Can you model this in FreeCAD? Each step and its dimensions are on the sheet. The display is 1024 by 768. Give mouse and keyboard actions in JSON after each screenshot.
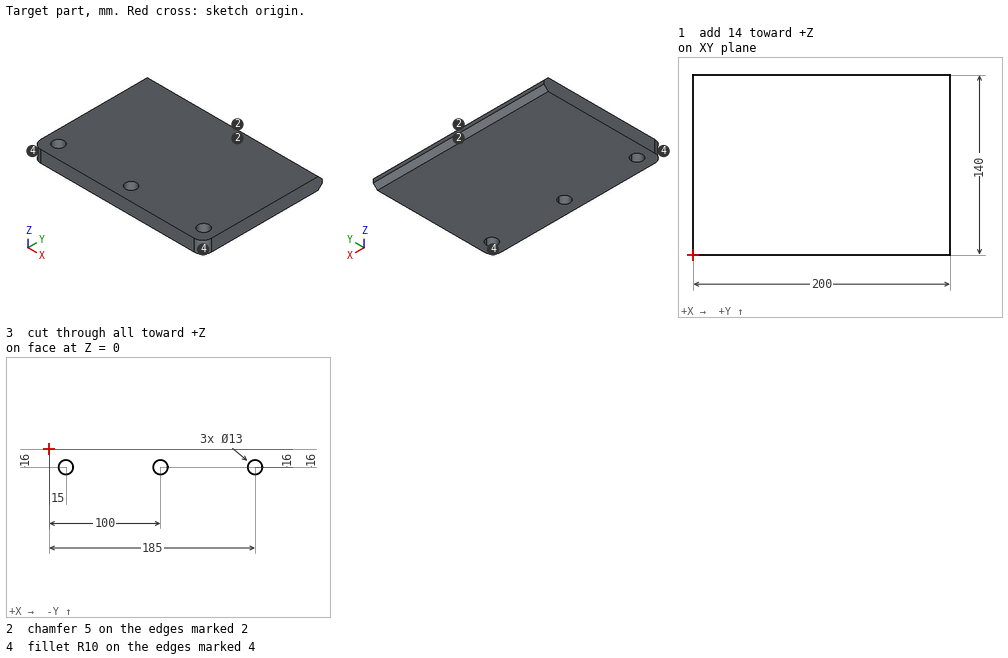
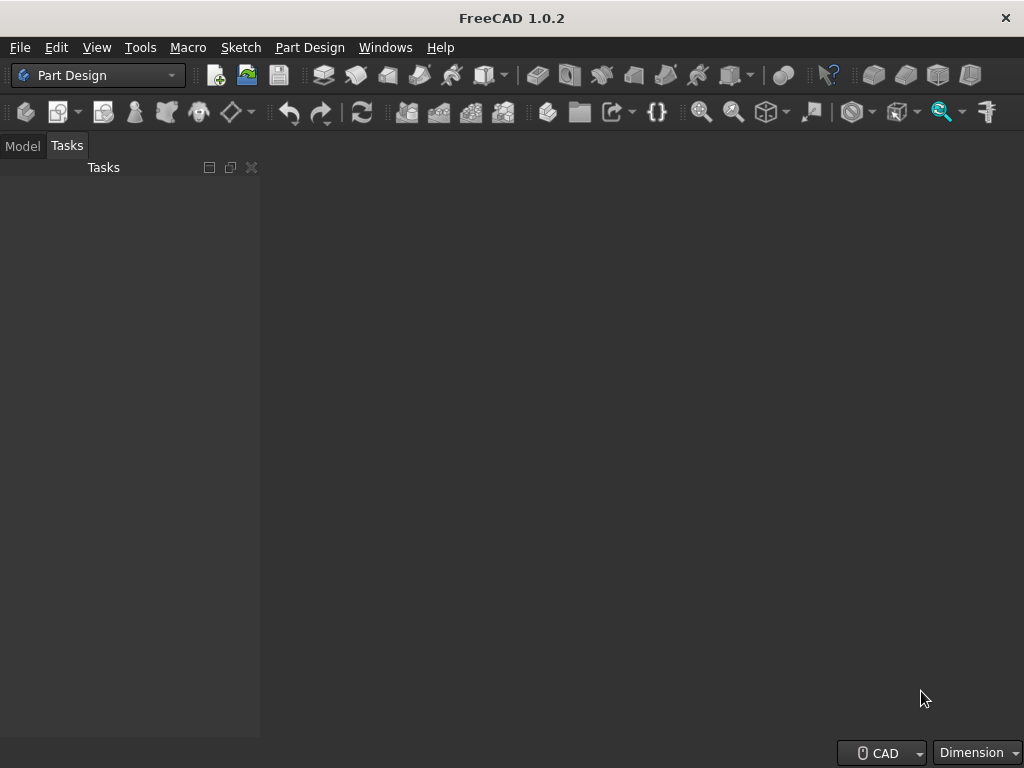
{"action": "left_click", "coordinate": [216, 76]}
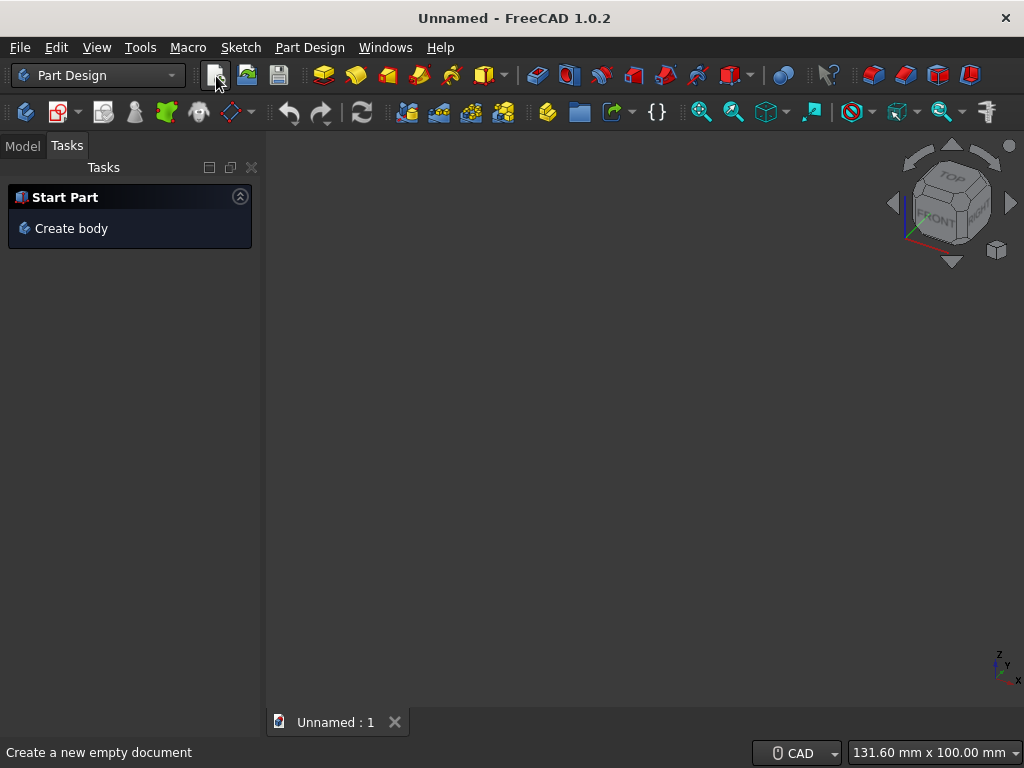
{"action": "left_click", "coordinate": [58, 112]}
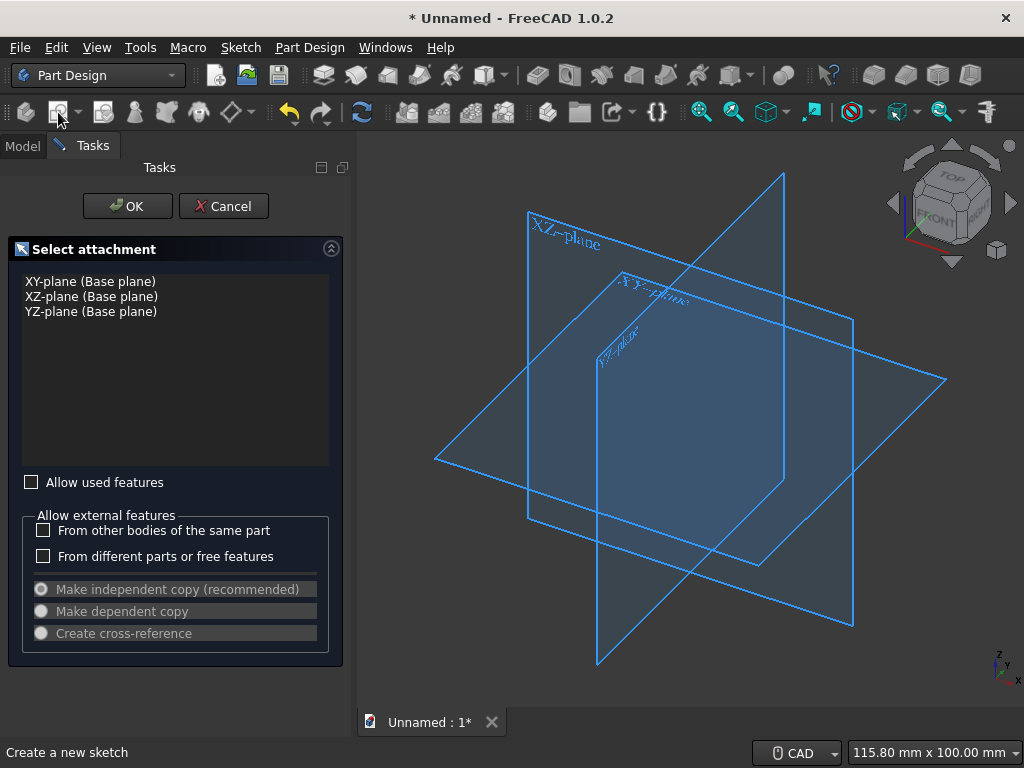
{"action": "left_click", "coordinate": [82, 282]}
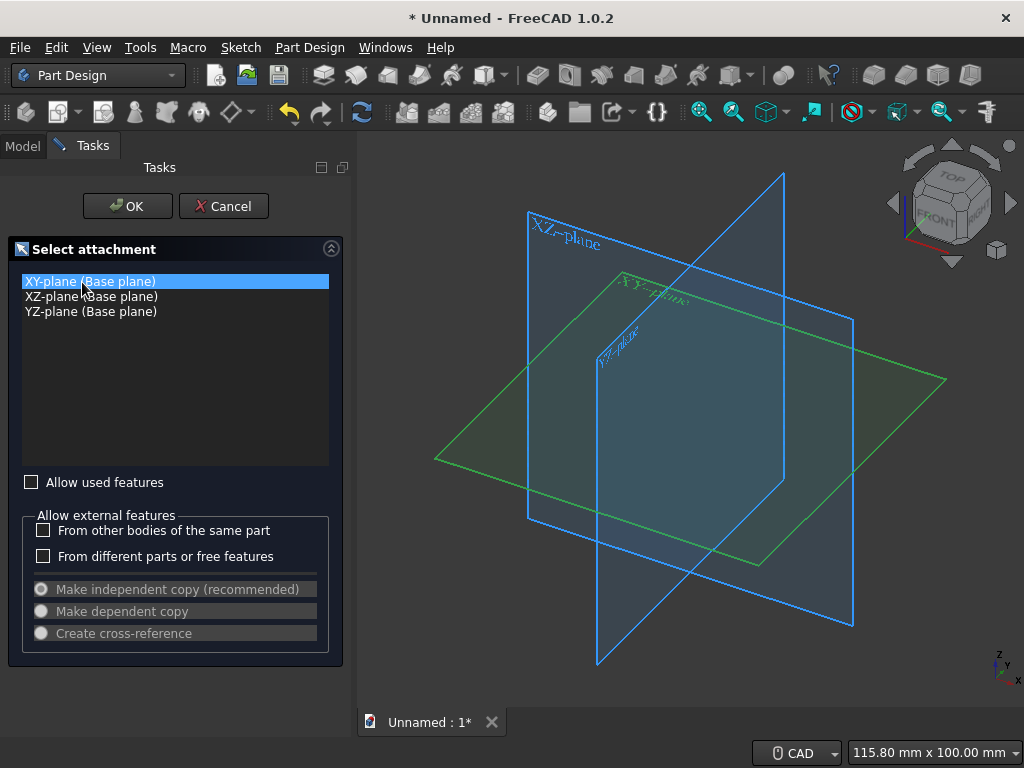
{"action": "left_click", "coordinate": [128, 206]}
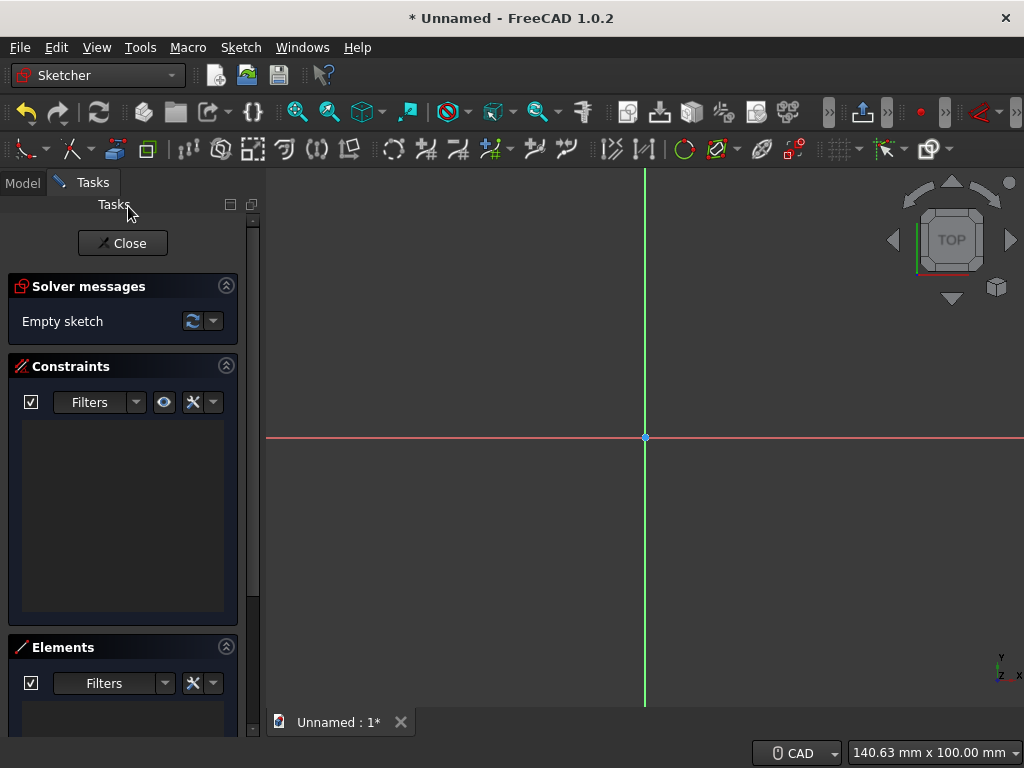
{"action": "scroll", "coordinate": [294, 657], "scroll_direction": "down", "scroll_amount": 5}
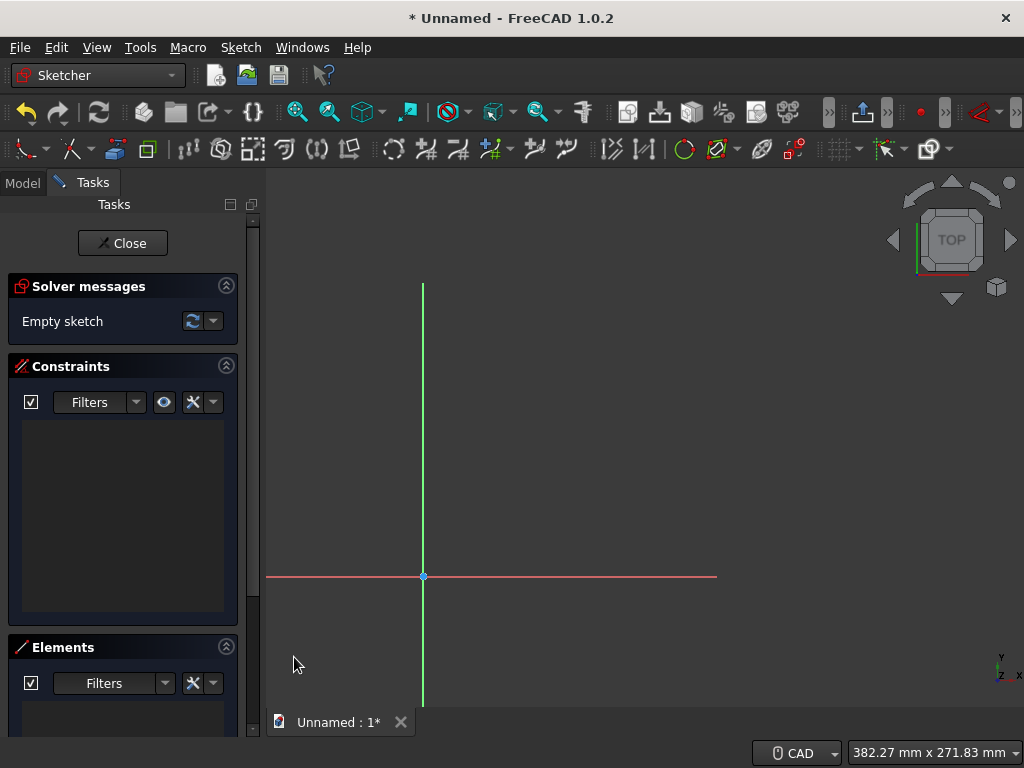
{"action": "key", "text": "g r"}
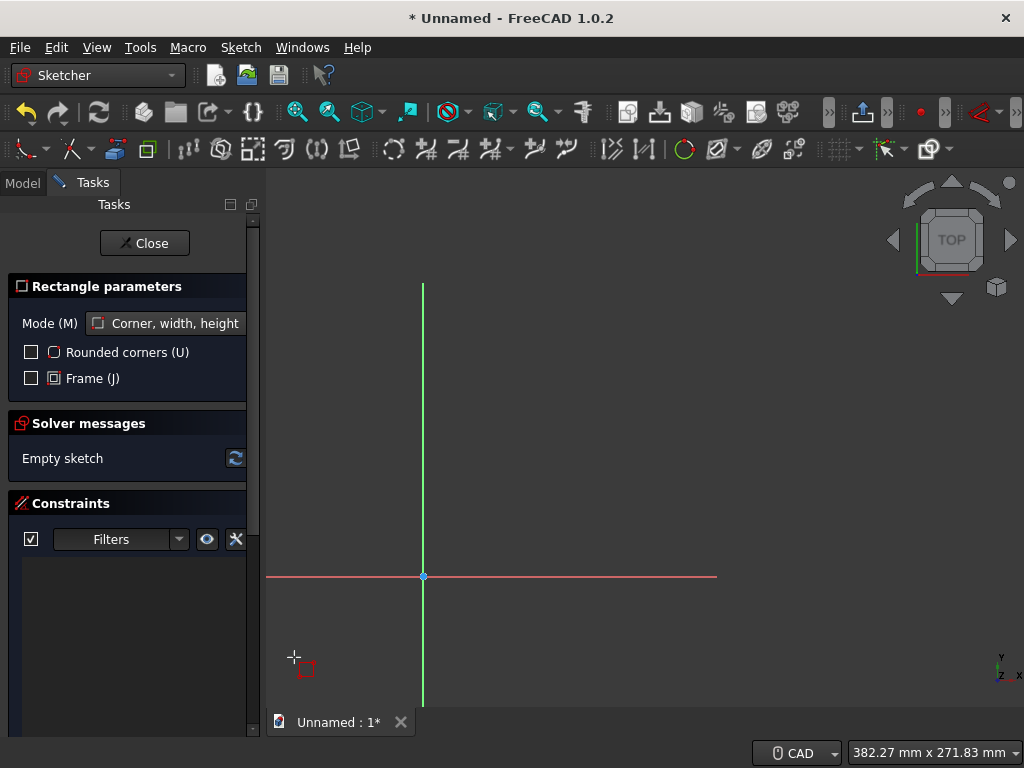
{"action": "left_click", "coordinate": [423, 577]}
{"action": "left_click", "coordinate": [820, 299]}
{"action": "key", "text": "Escape"}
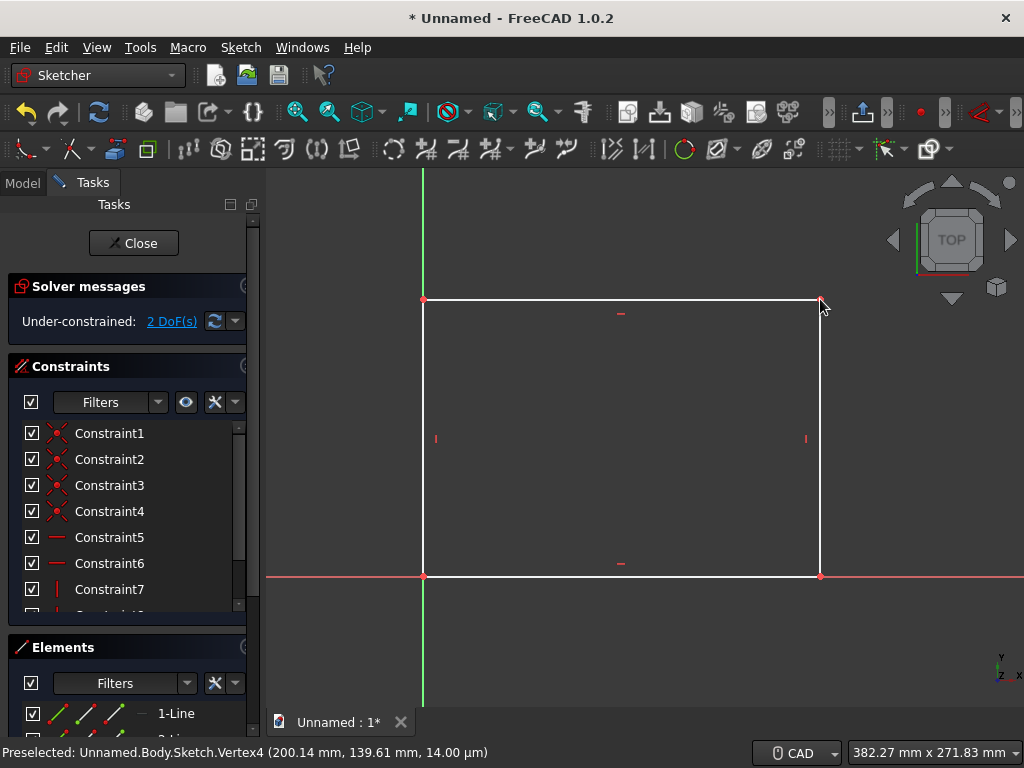
{"action": "left_click", "coordinate": [980, 112]}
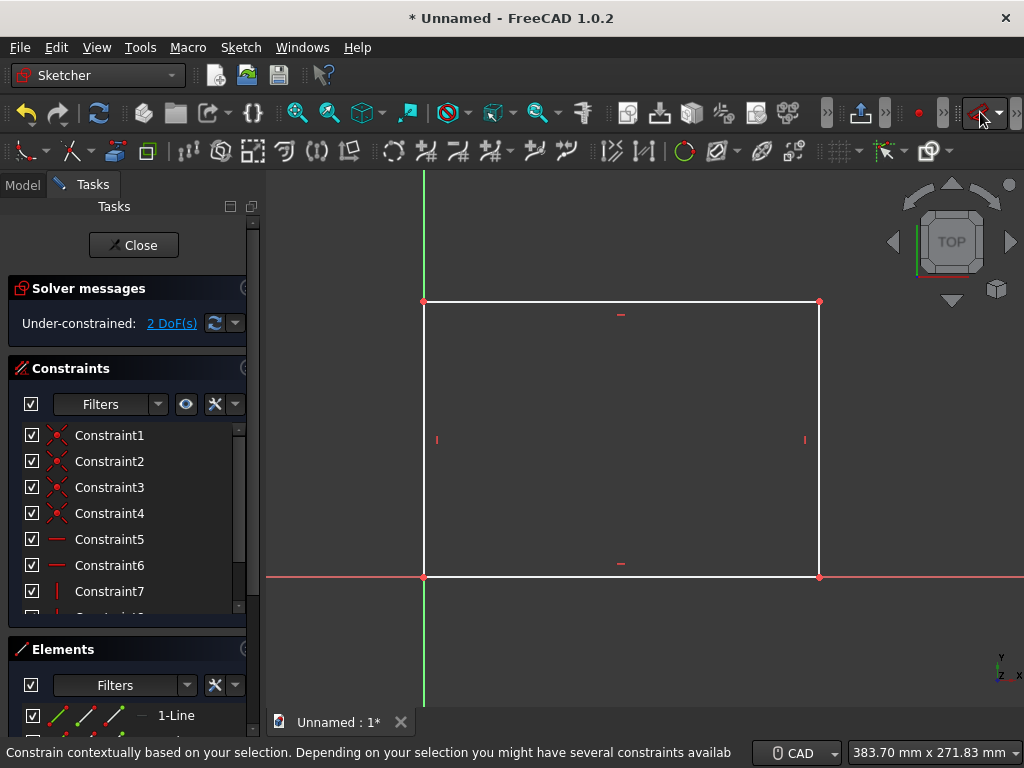
{"action": "left_click", "coordinate": [543, 577]}
{"action": "left_click", "coordinate": [622, 611]}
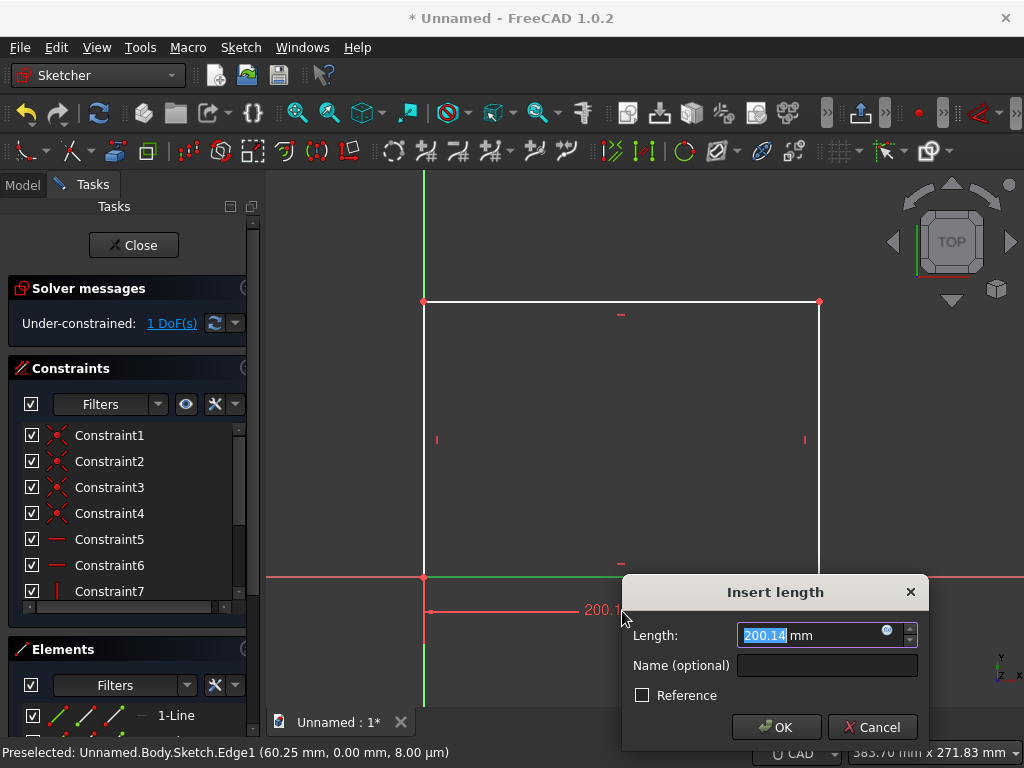
{"action": "type", "text": "200"}
{"action": "key", "text": "Return"}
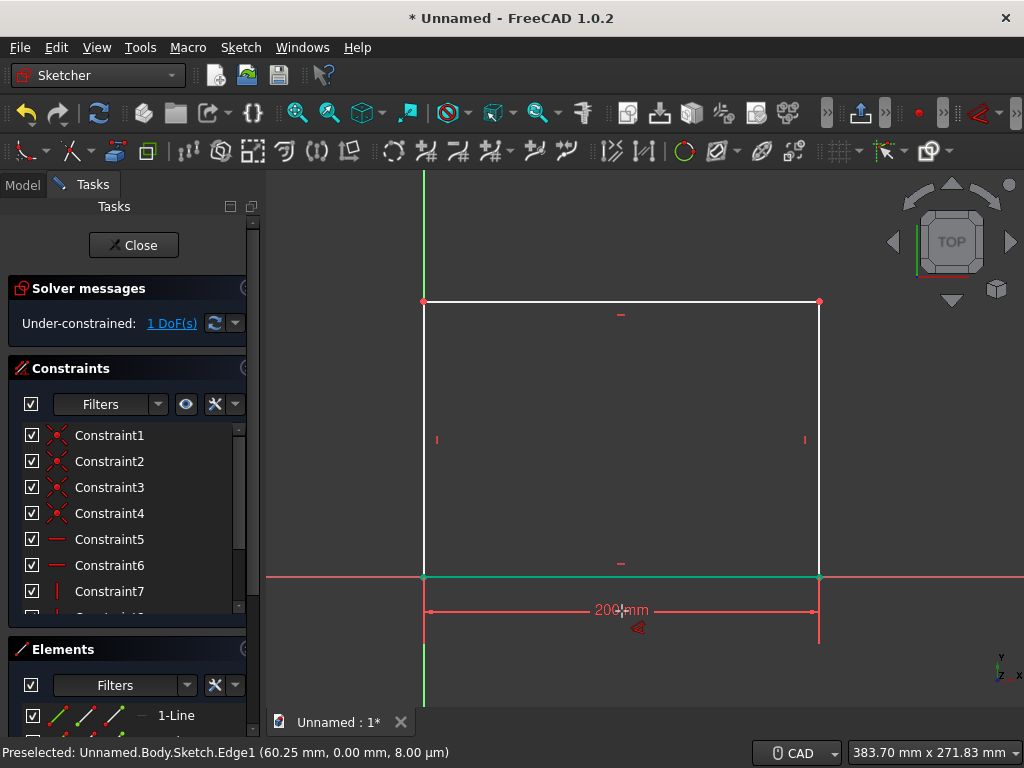
{"action": "left_click", "coordinate": [819, 495]}
{"action": "left_click", "coordinate": [853, 439]}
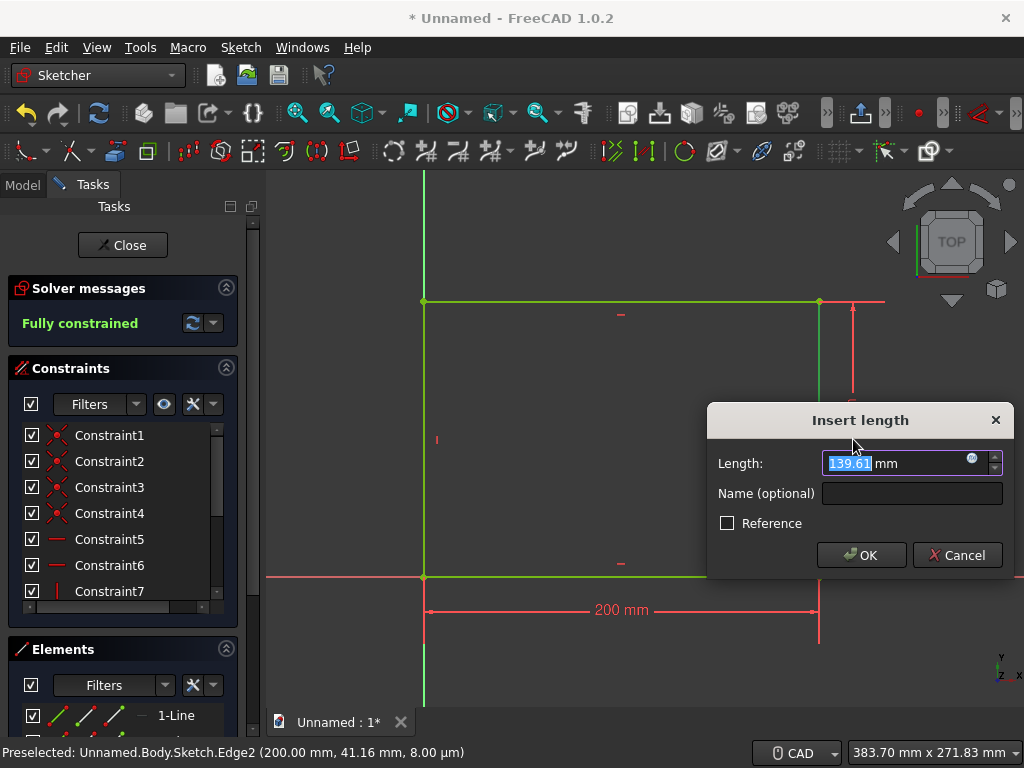
{"action": "type", "text": "140"}
{"action": "key", "text": "Return"}
{"action": "key", "text": "Escape"}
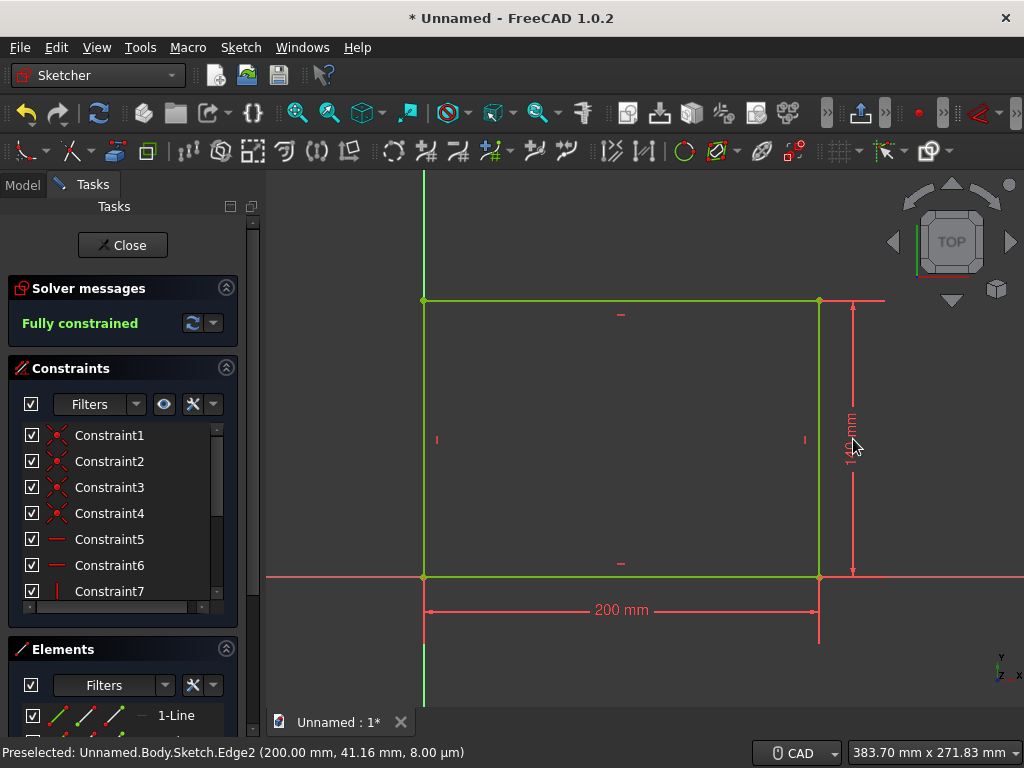
{"action": "left_click", "coordinate": [123, 245]}